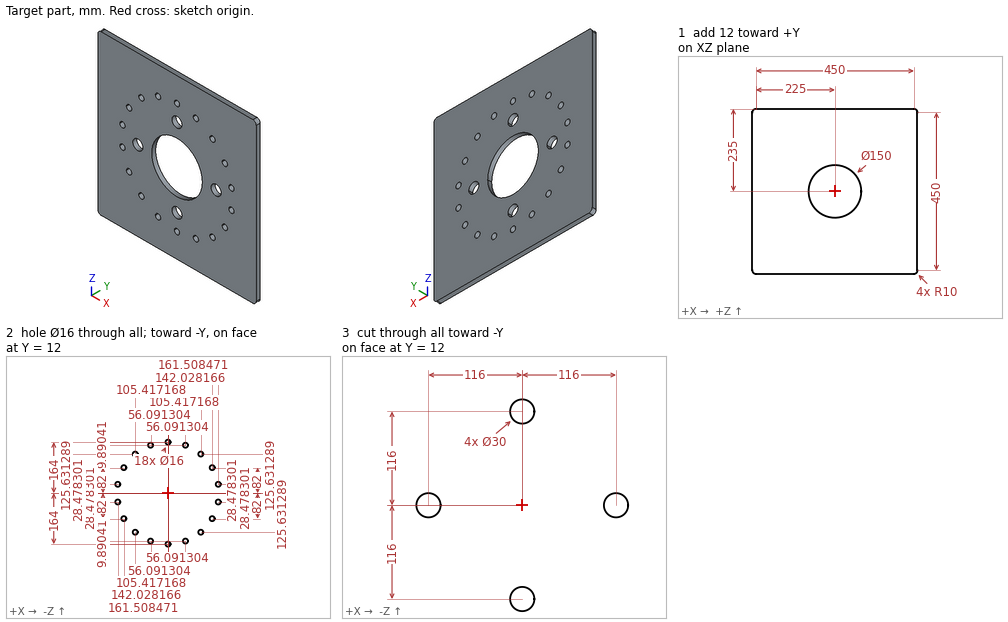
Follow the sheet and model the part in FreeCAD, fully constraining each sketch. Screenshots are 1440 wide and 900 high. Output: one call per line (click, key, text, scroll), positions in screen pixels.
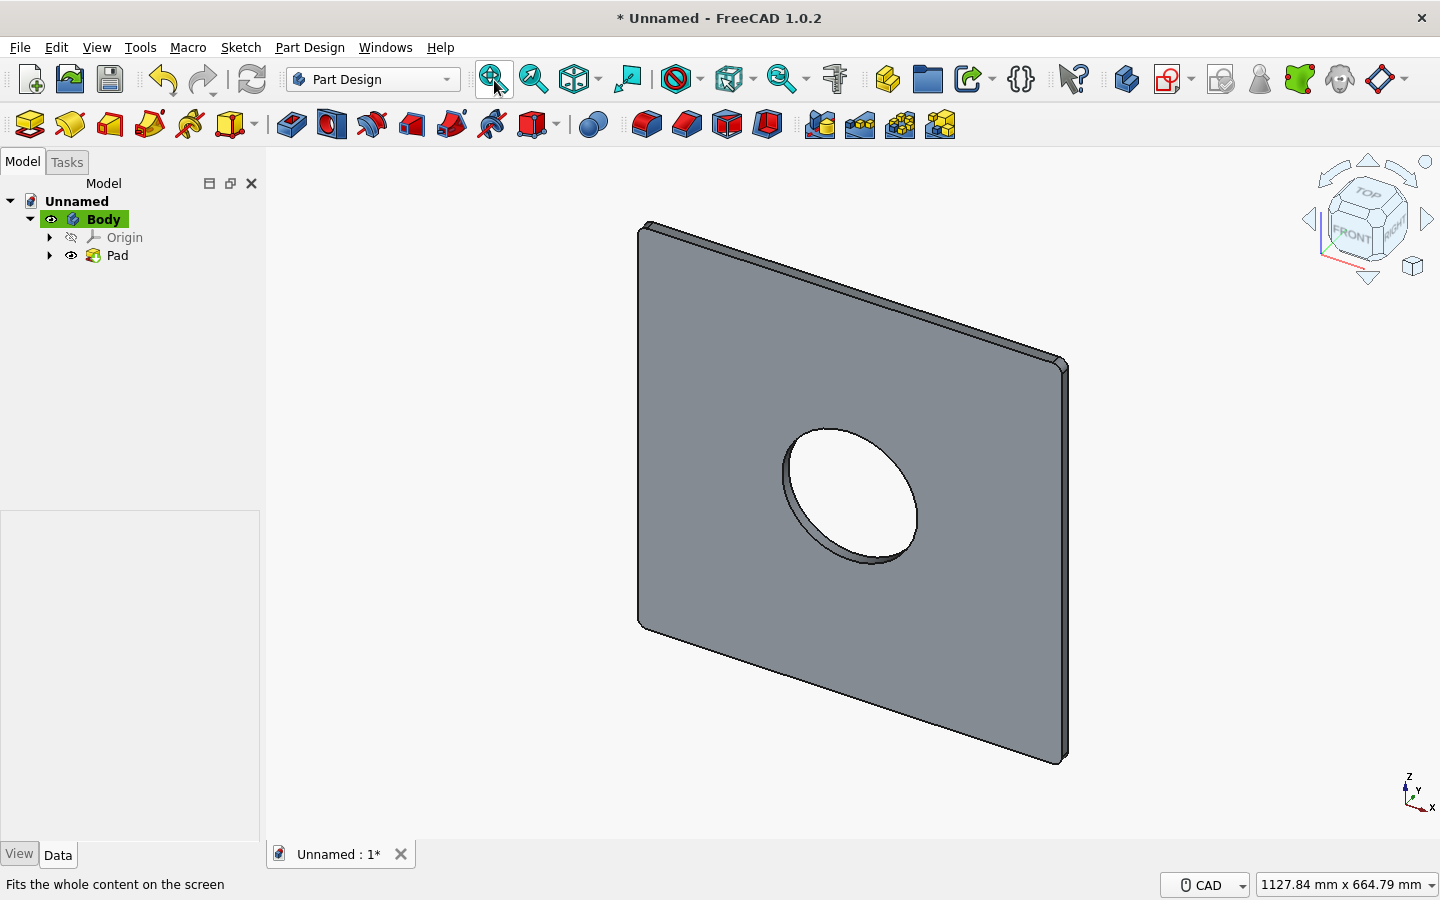
key(4)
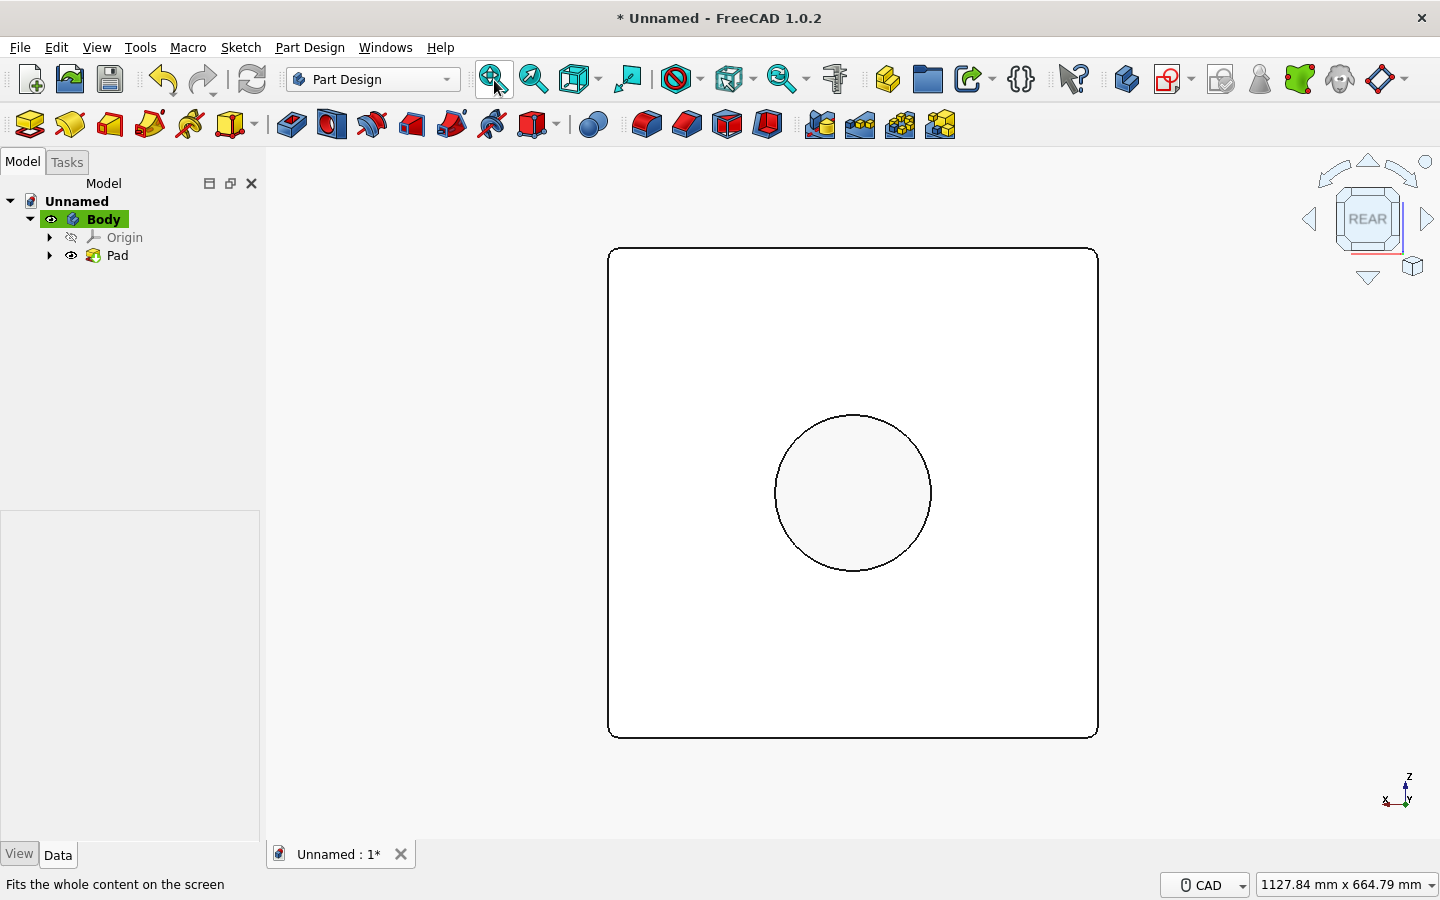
click(713, 632)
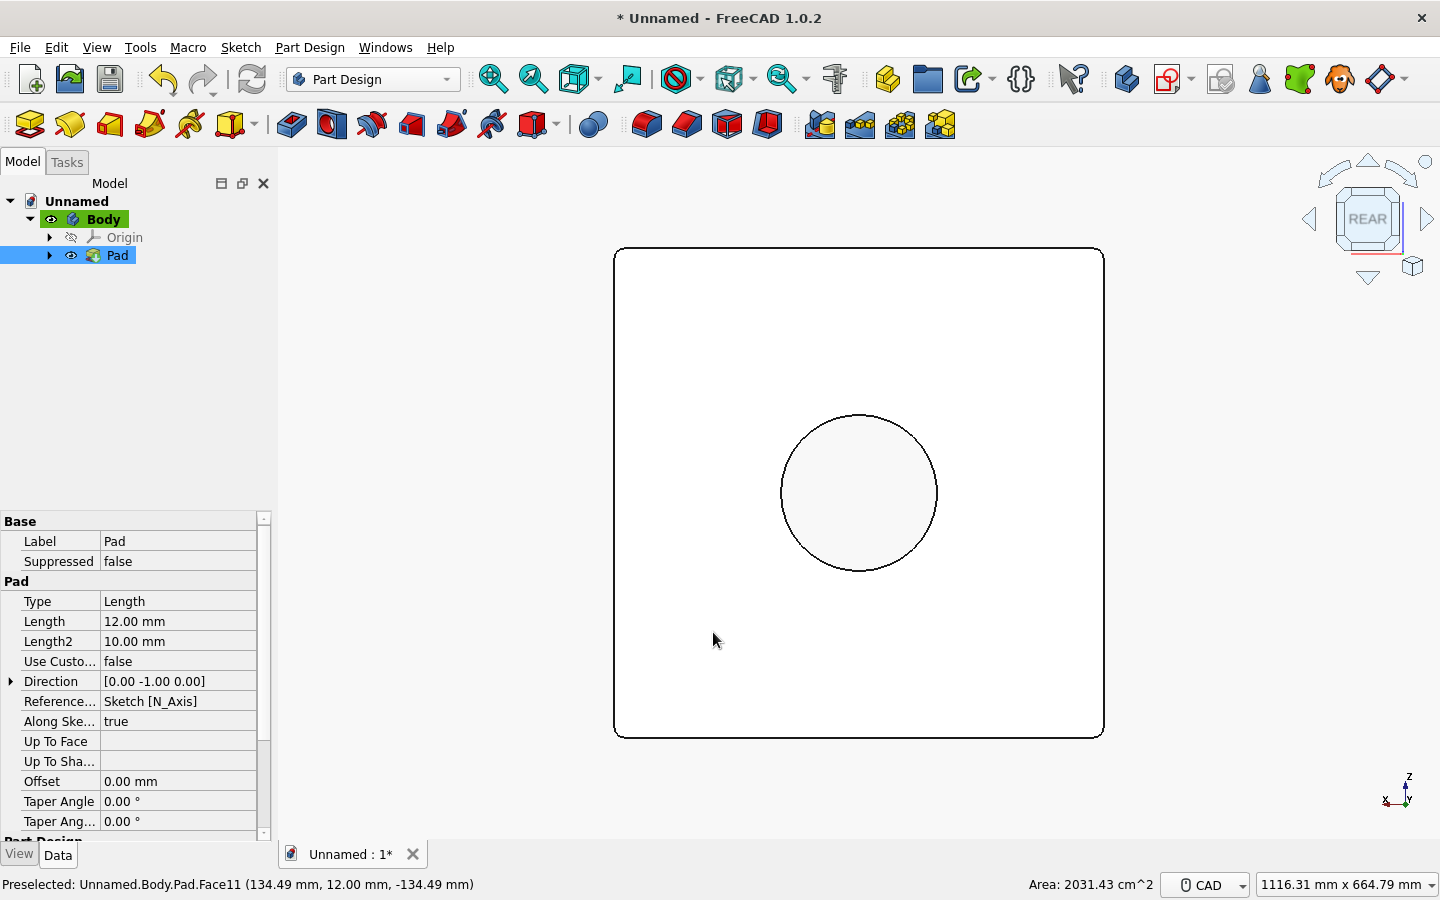
click(1168, 80)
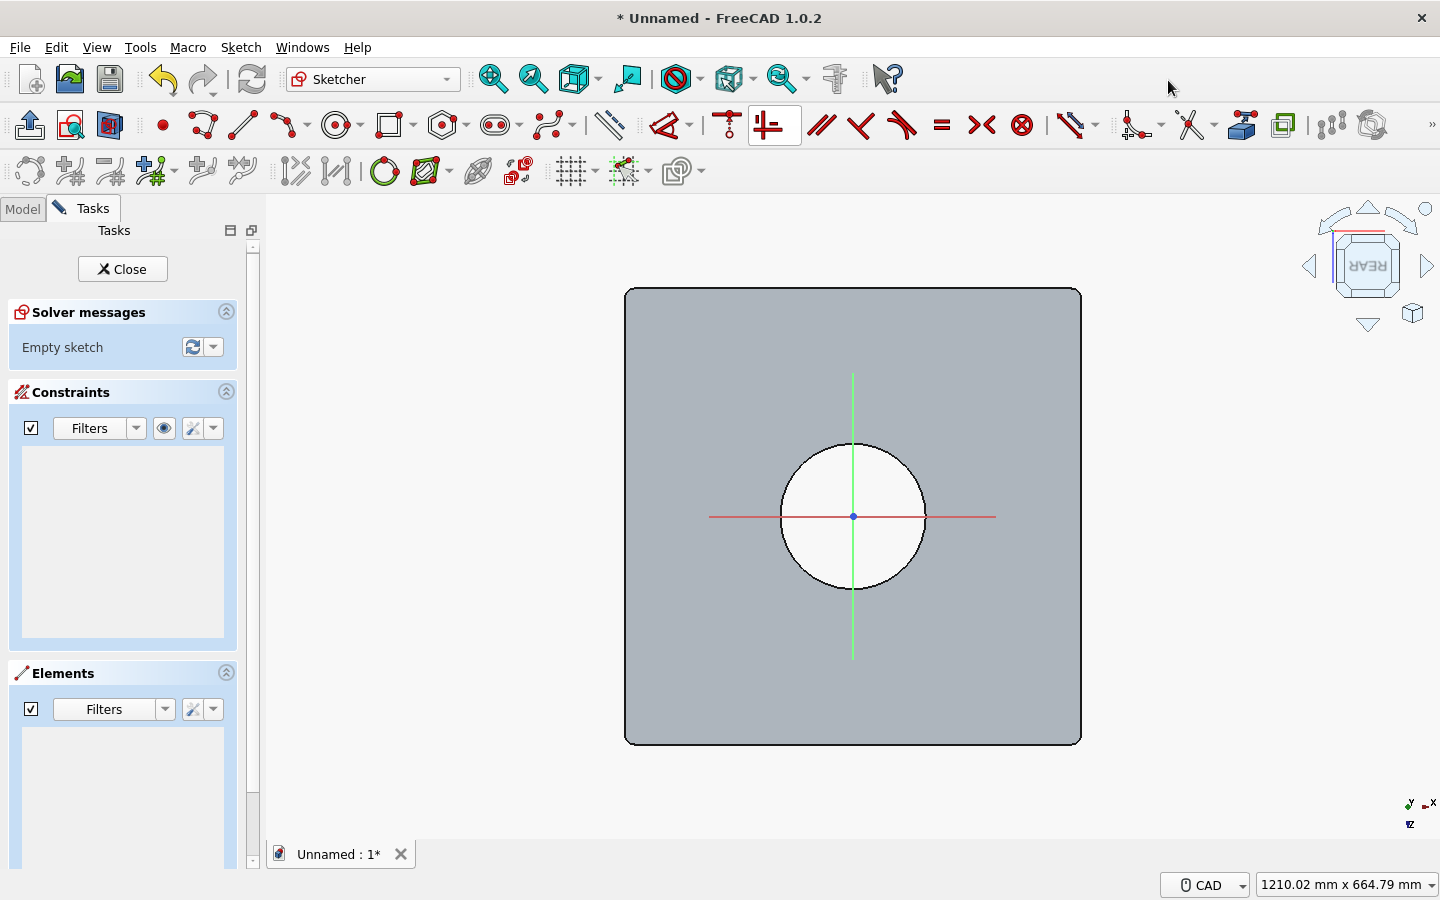
key(g)
key(c)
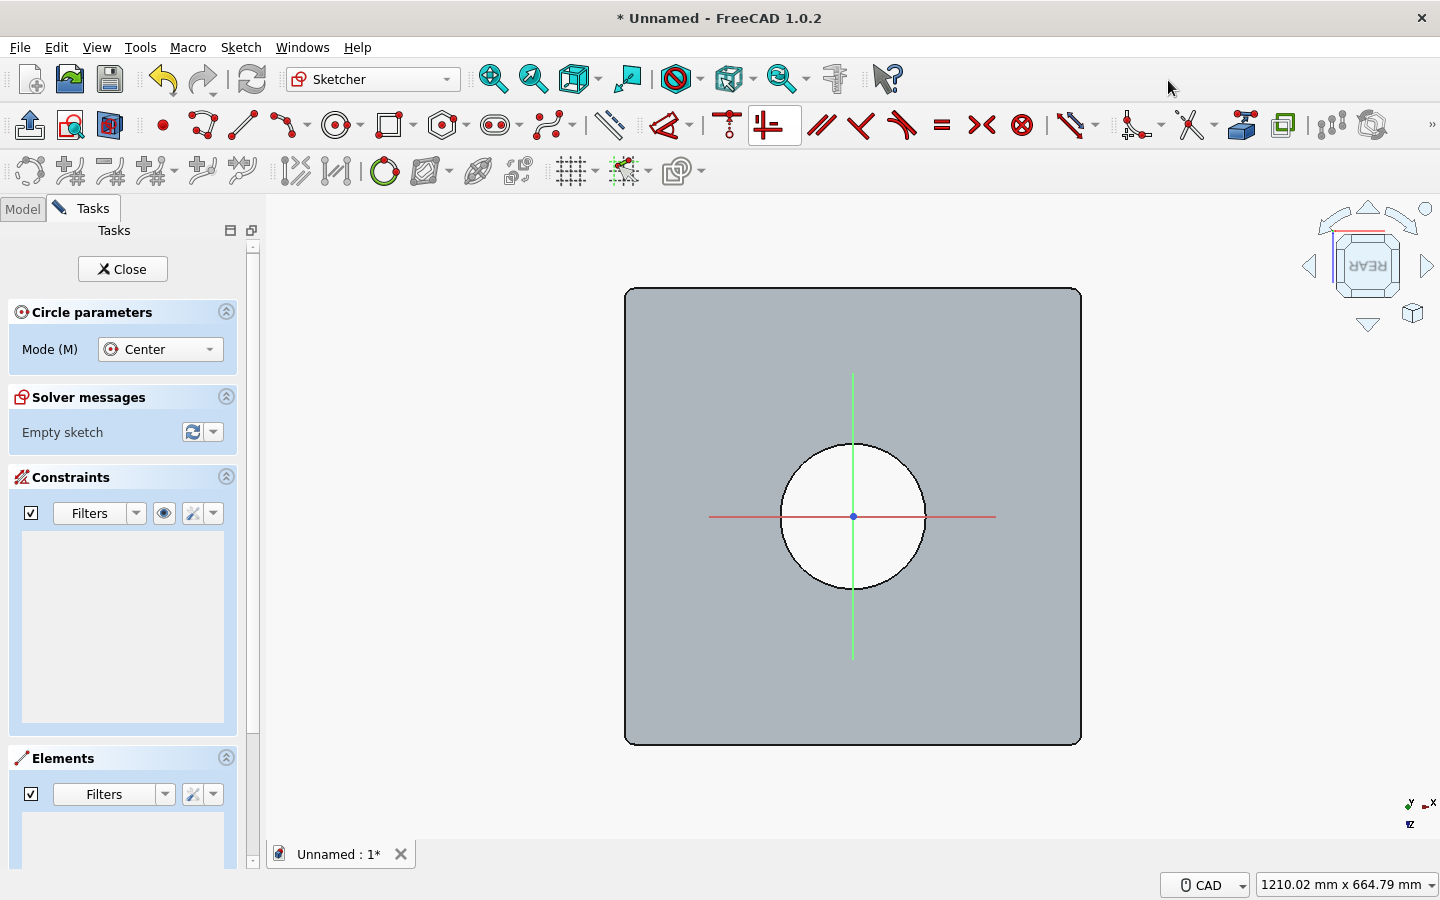
scroll(853, 357, up, 6)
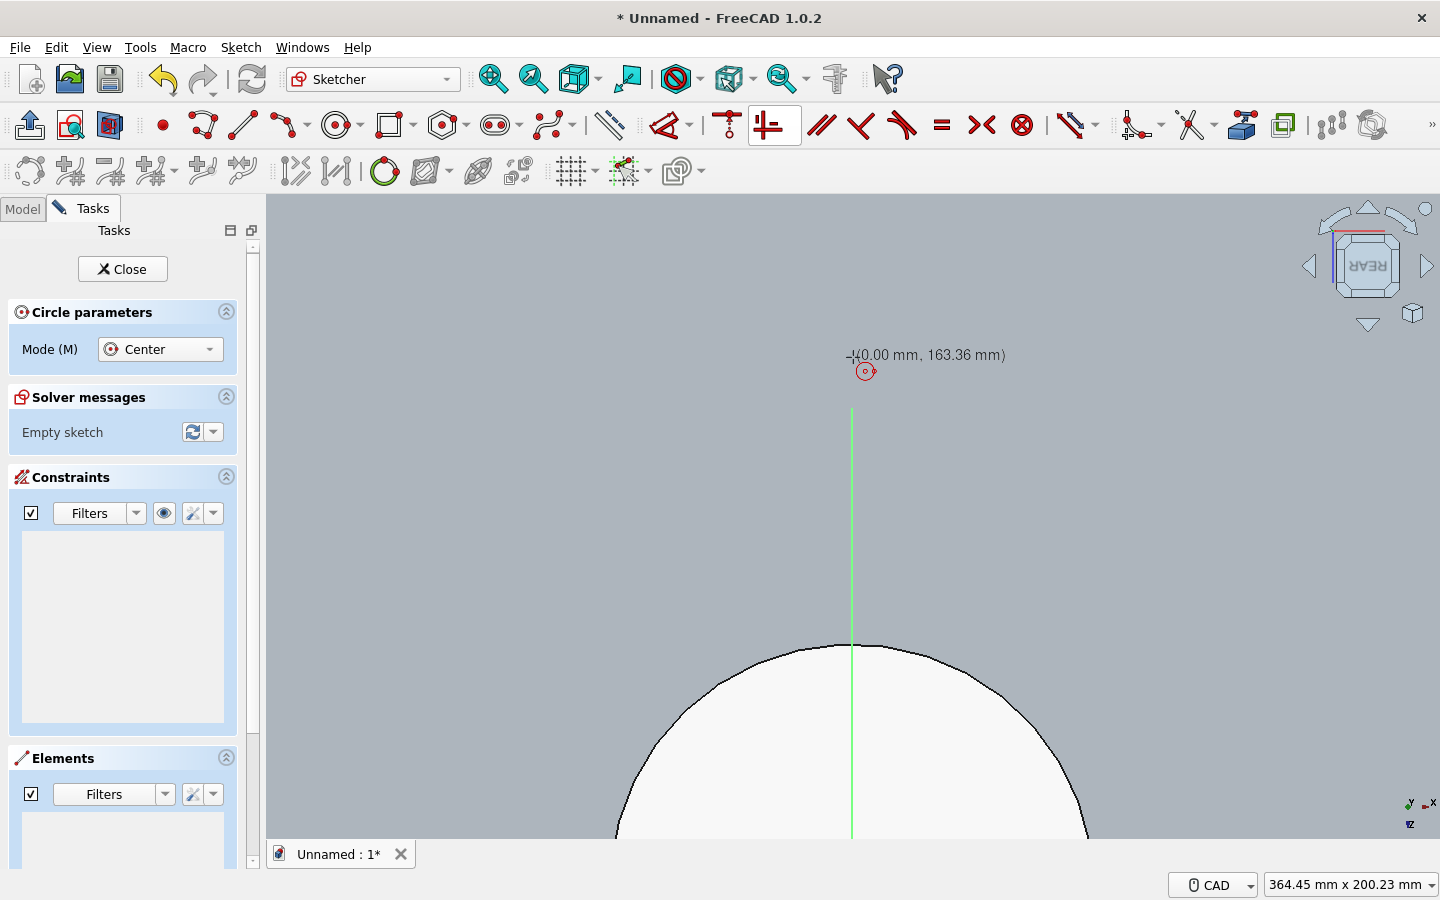
click(852, 358)
move(870, 339)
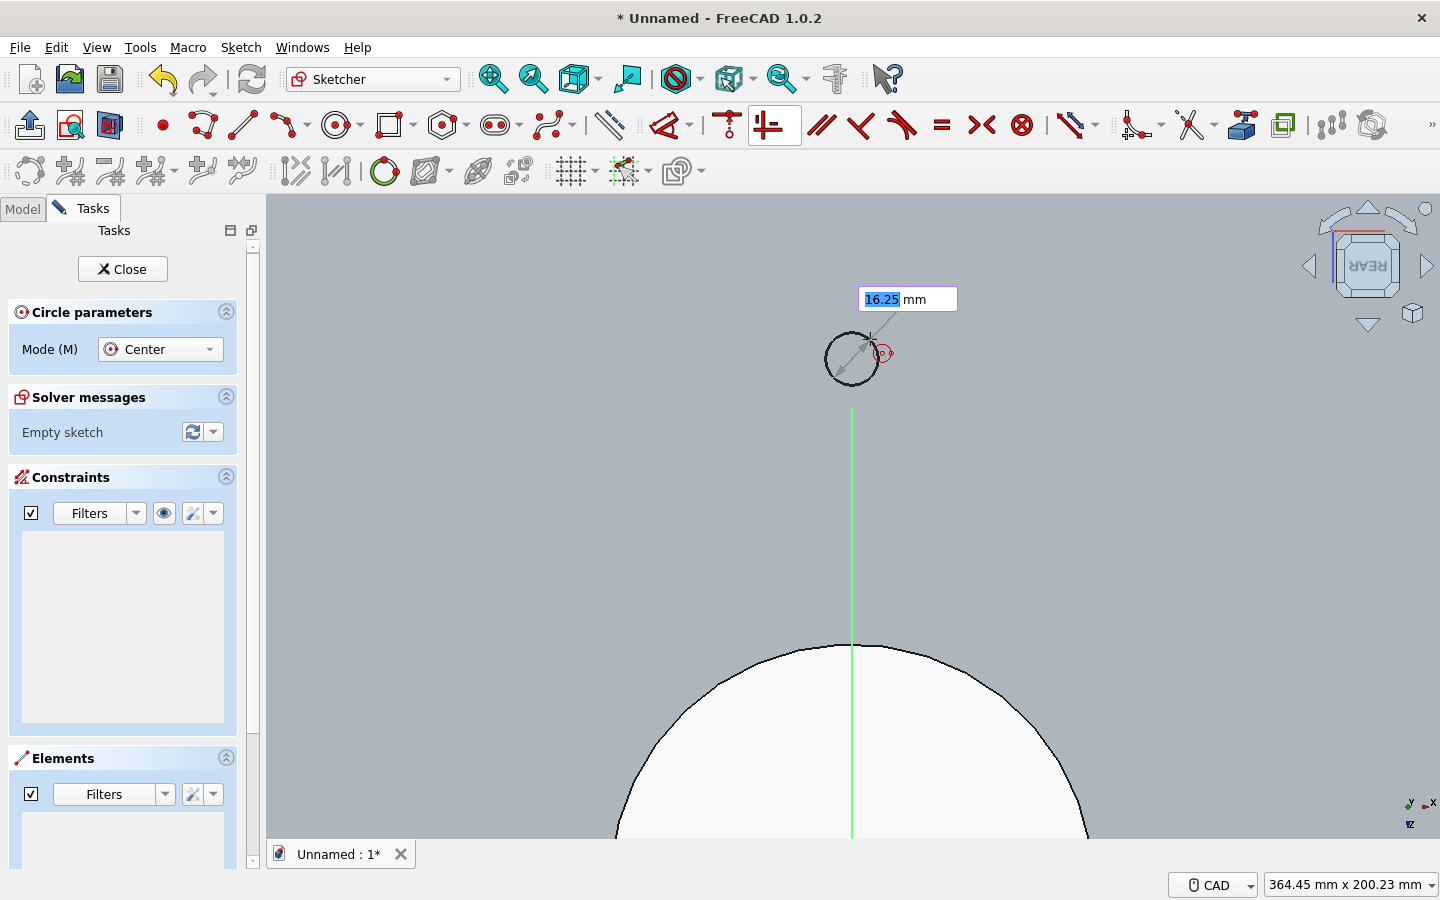
text(16)
key(Return)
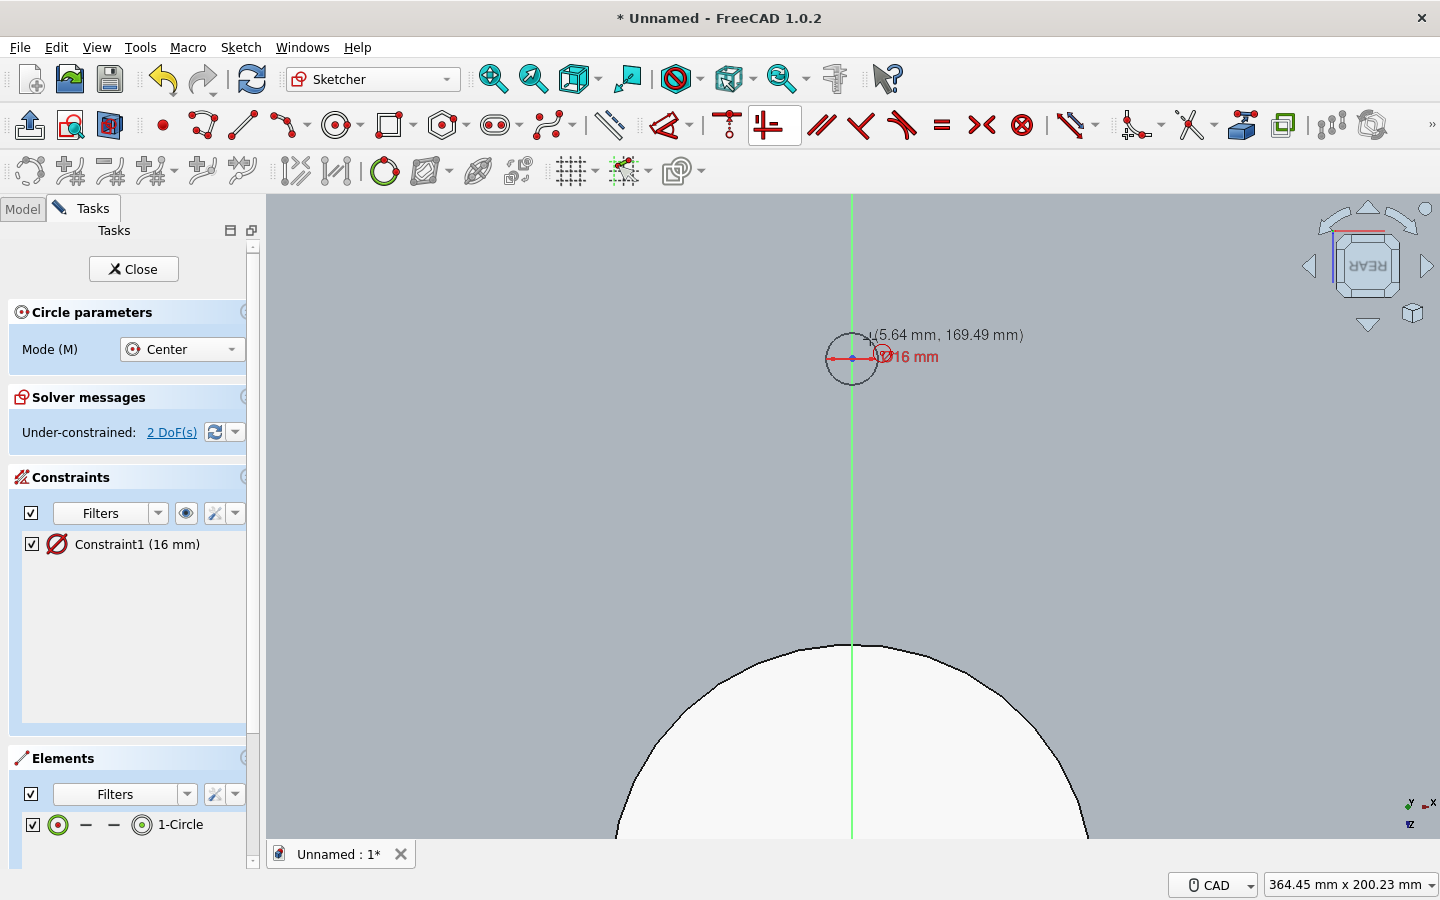
click(1033, 390)
move(1051, 371)